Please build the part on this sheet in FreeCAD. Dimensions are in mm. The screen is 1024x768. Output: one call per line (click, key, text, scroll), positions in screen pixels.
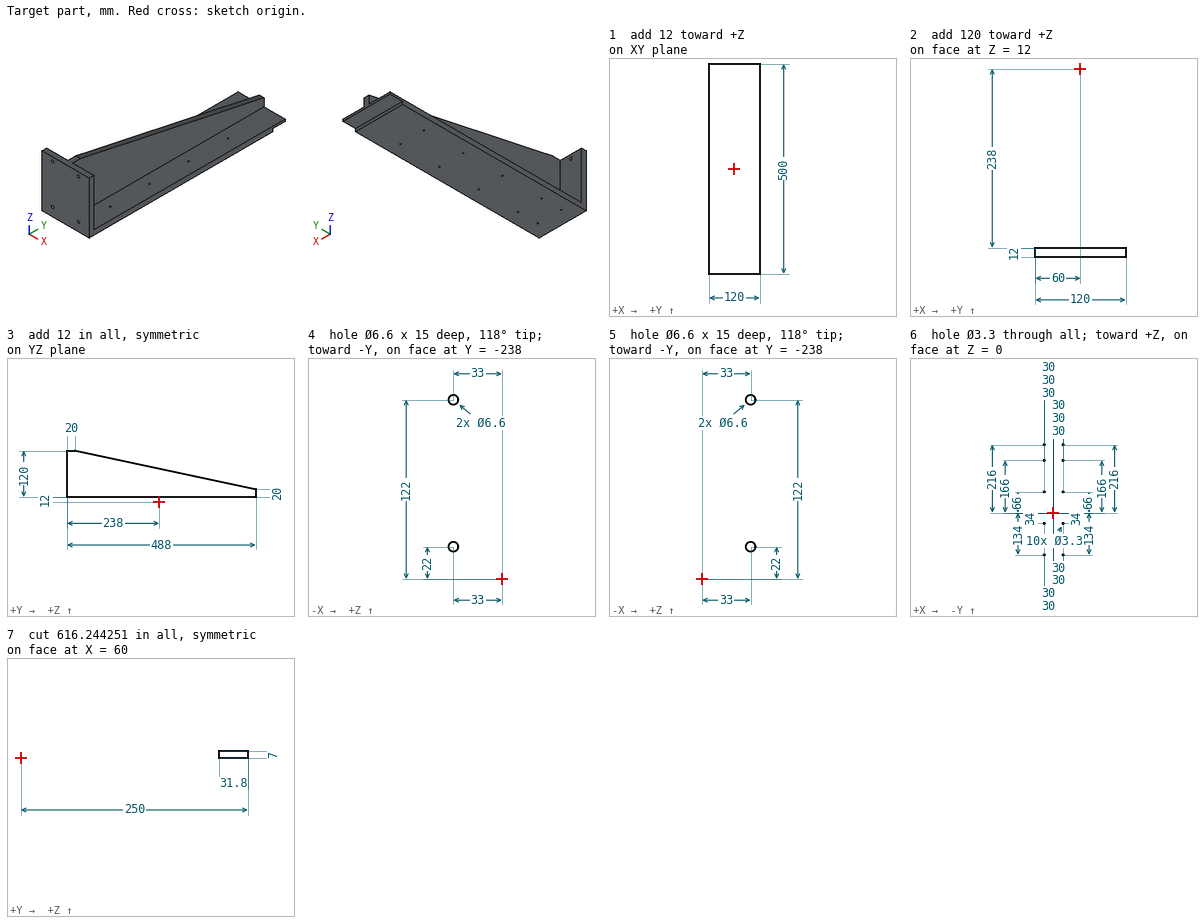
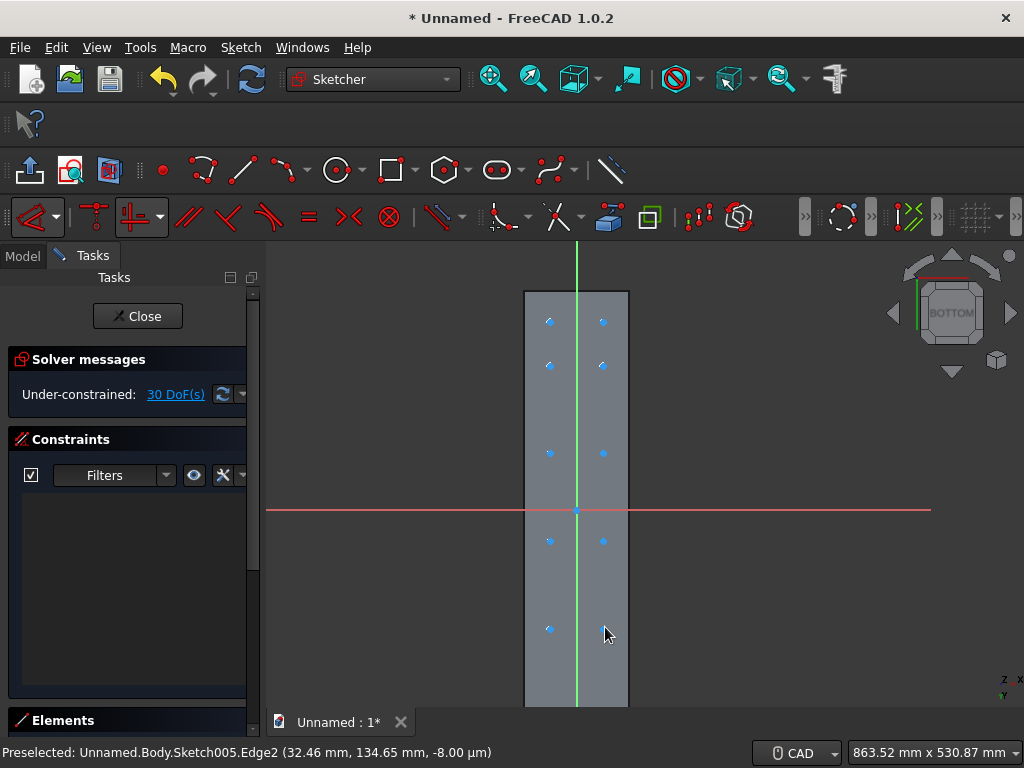
scroll(604, 452, up, 10)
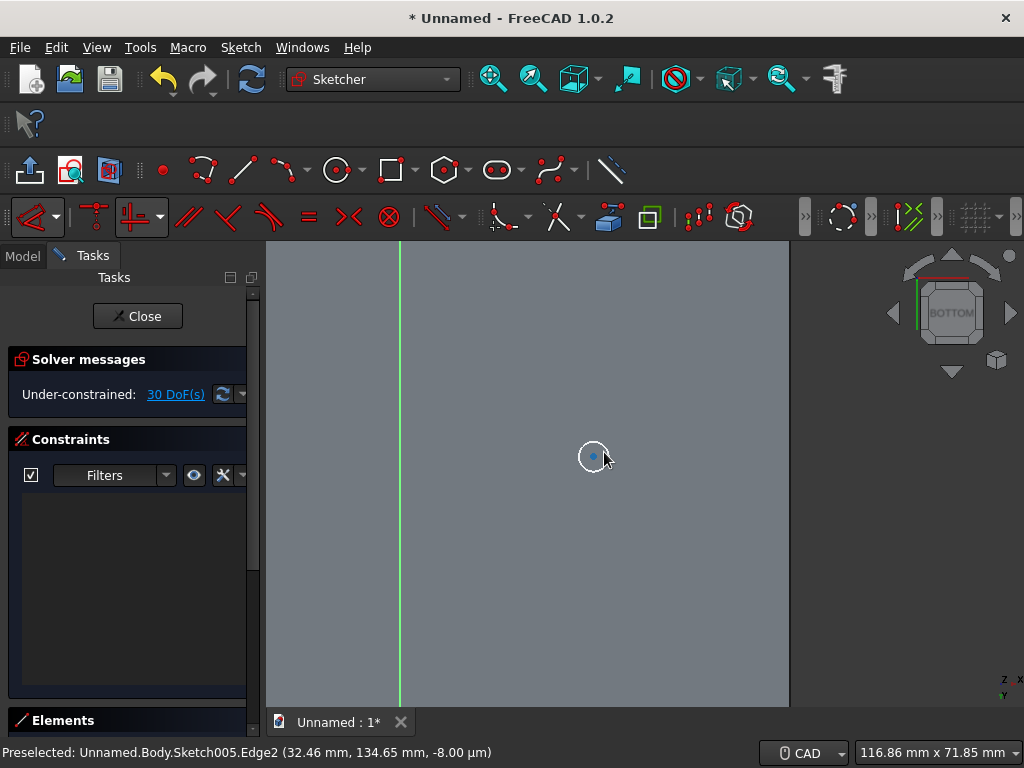
click(604, 446)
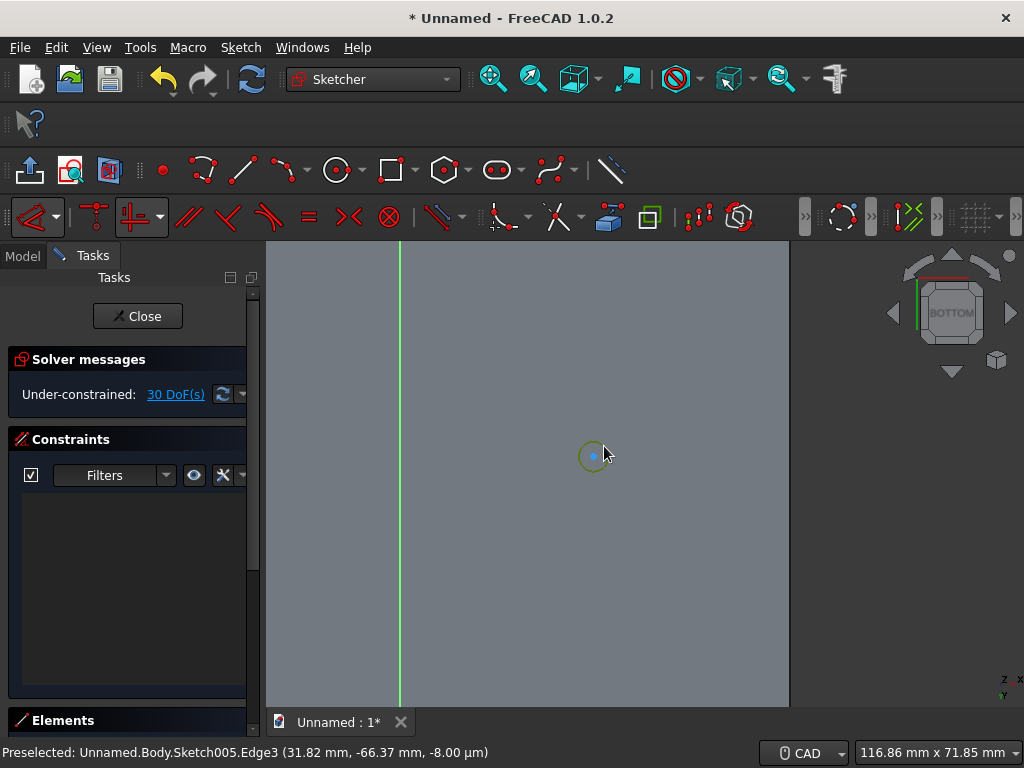
scroll(604, 452, down, 10)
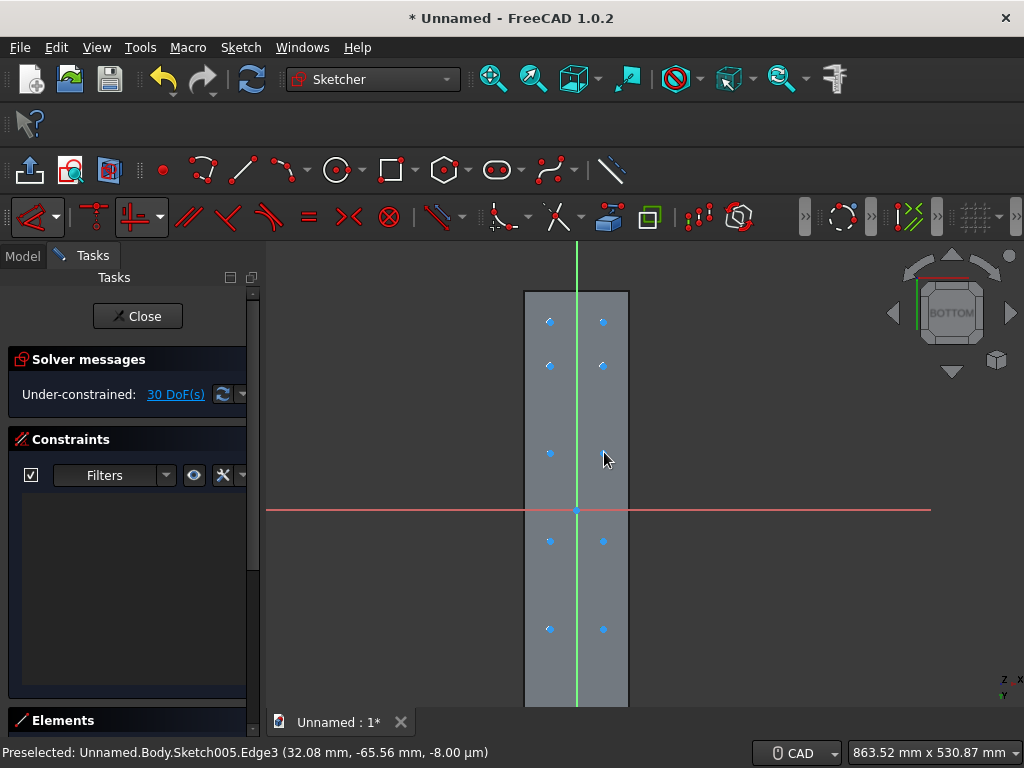
scroll(605, 364, up, 9)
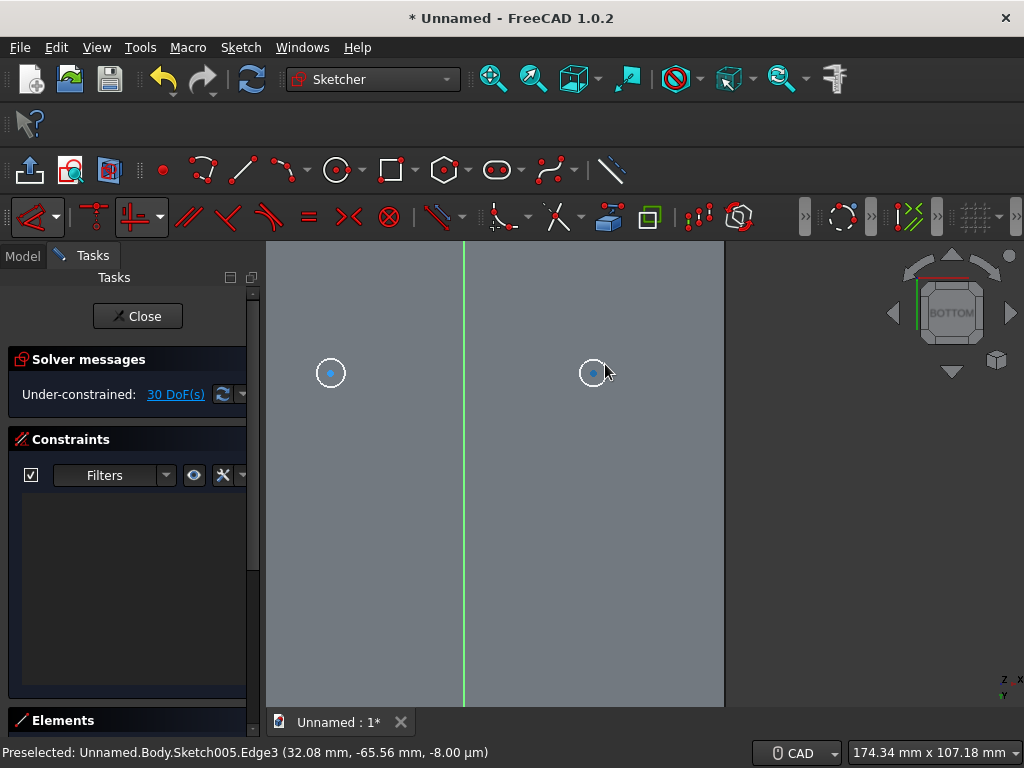
click(602, 363)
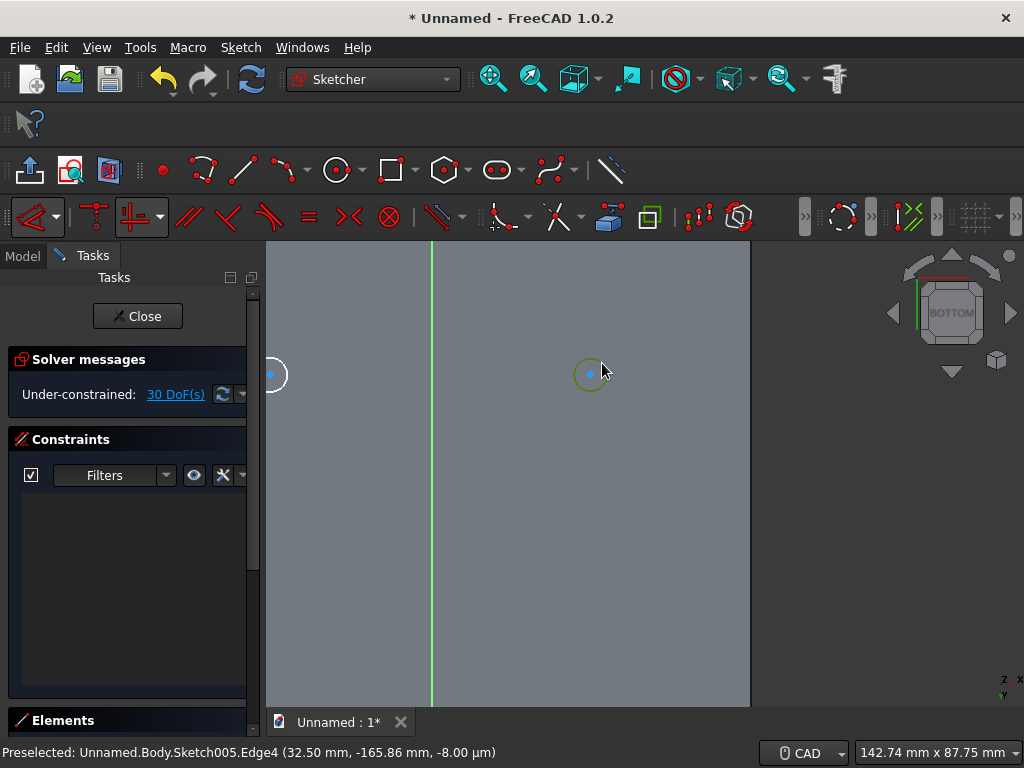
scroll(605, 364, down, 9)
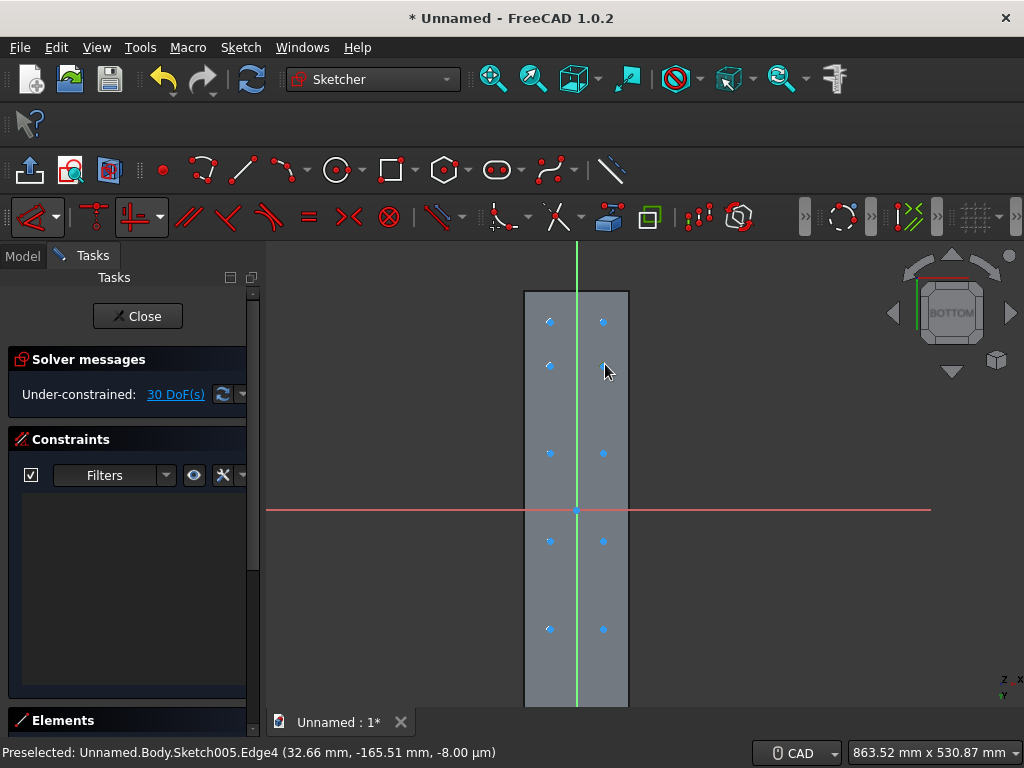
scroll(605, 320, up, 9)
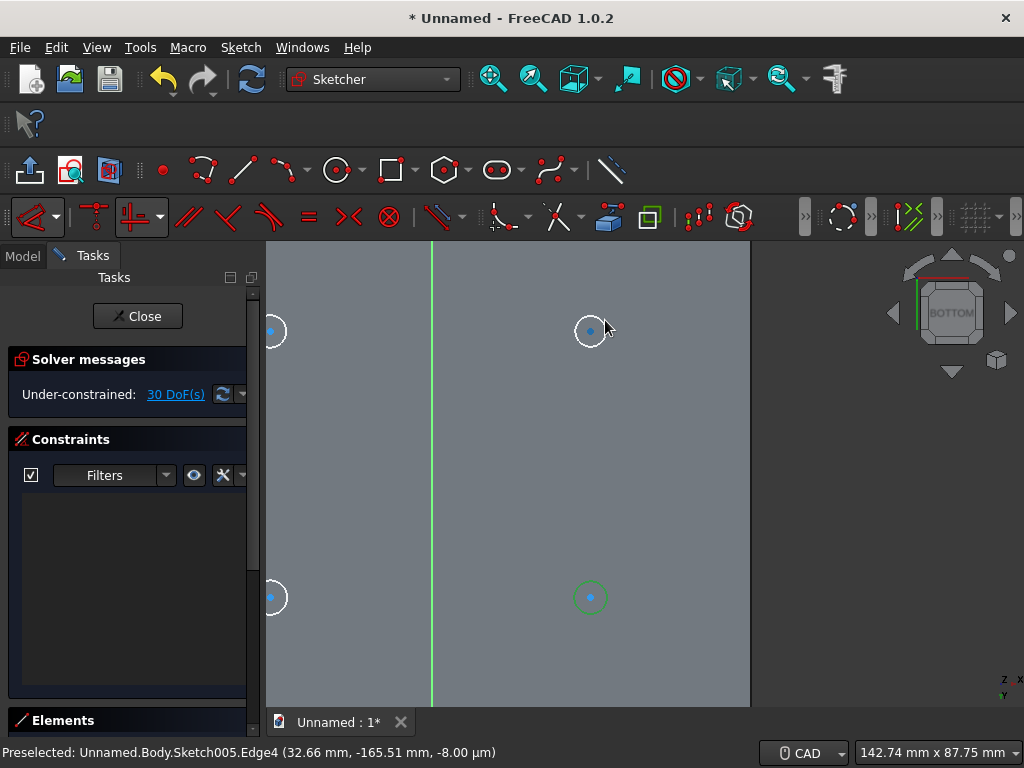
click(601, 321)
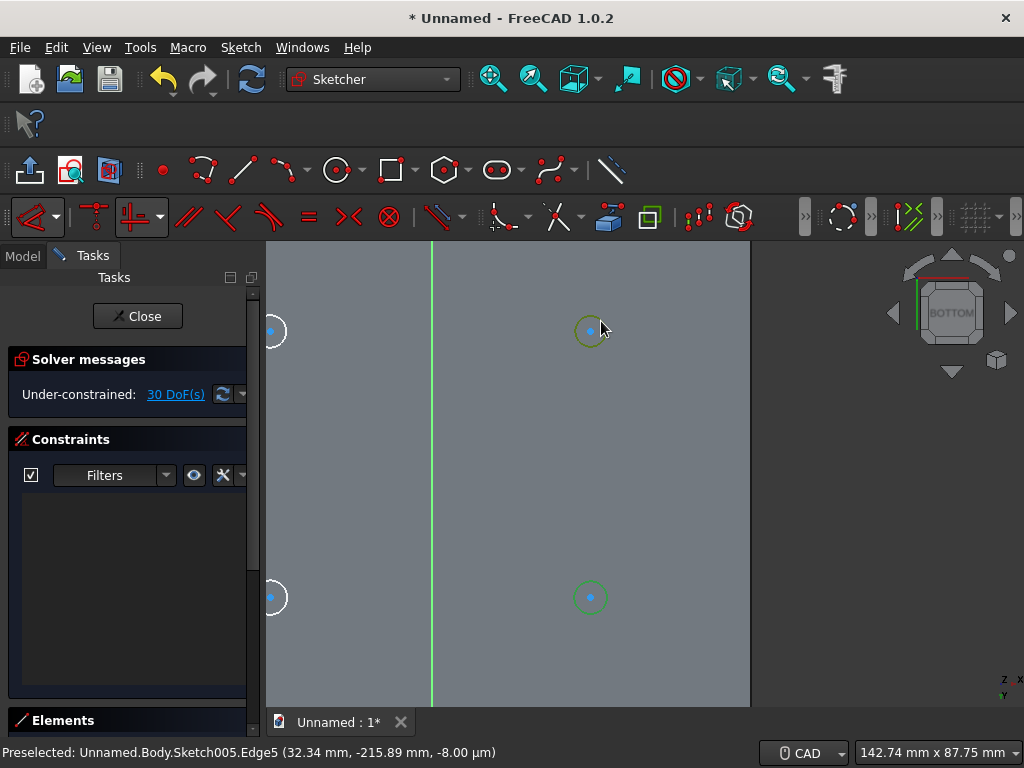
scroll(605, 320, down, 9)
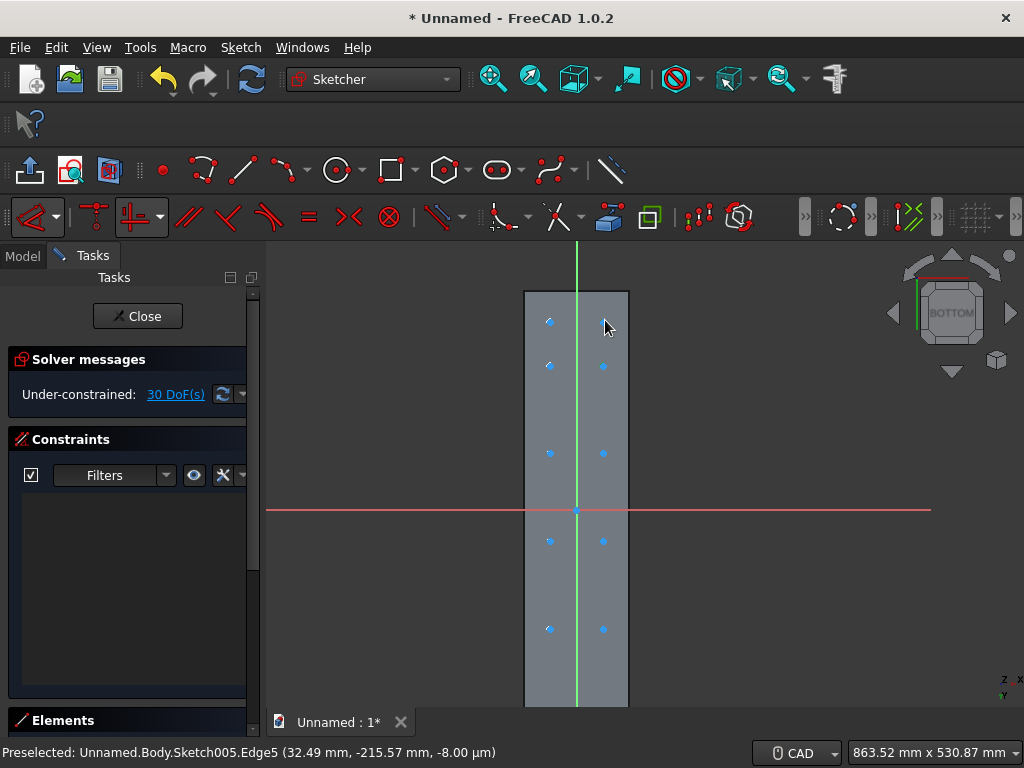
scroll(552, 320, up, 9)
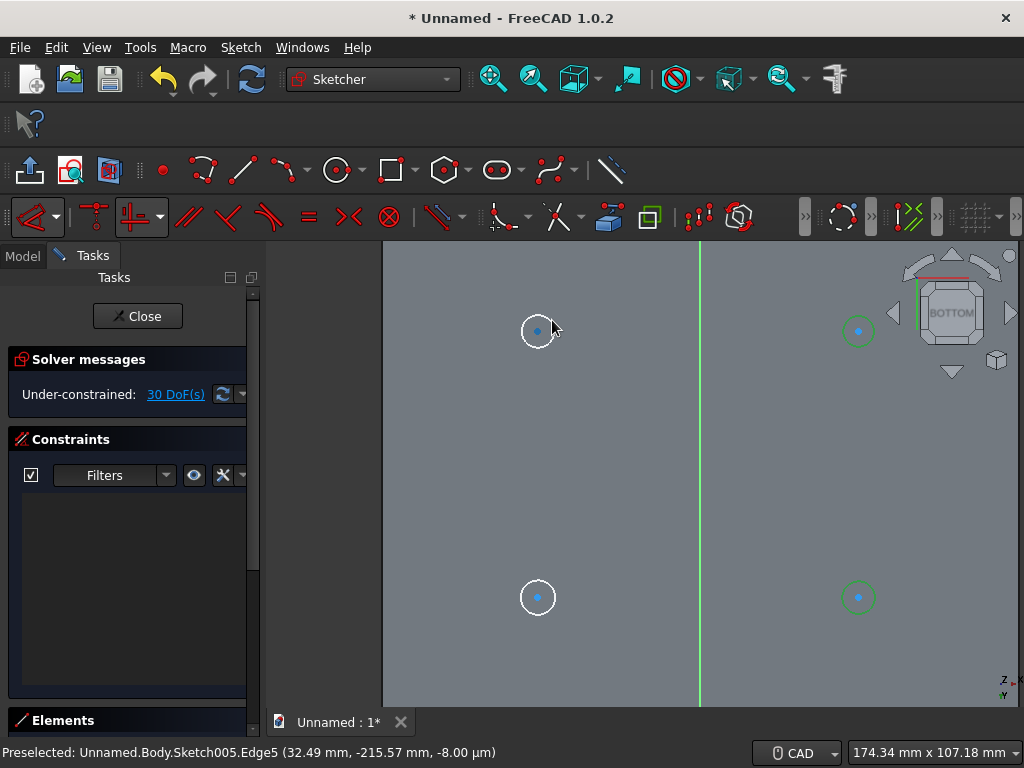
click(549, 320)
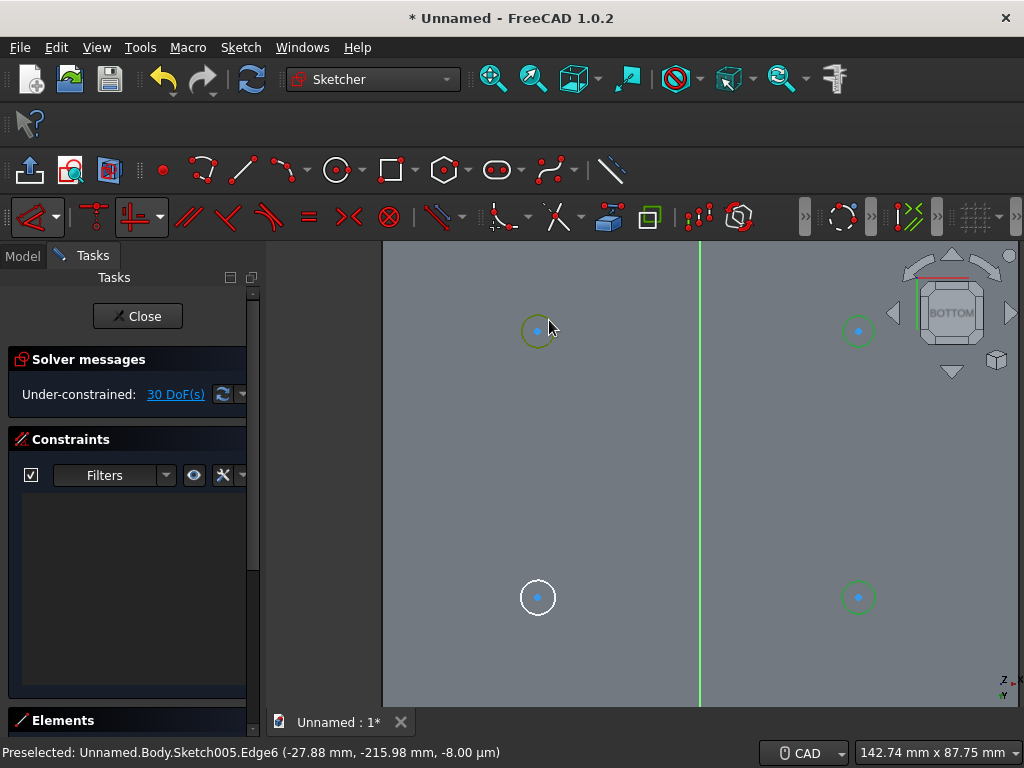
click(550, 585)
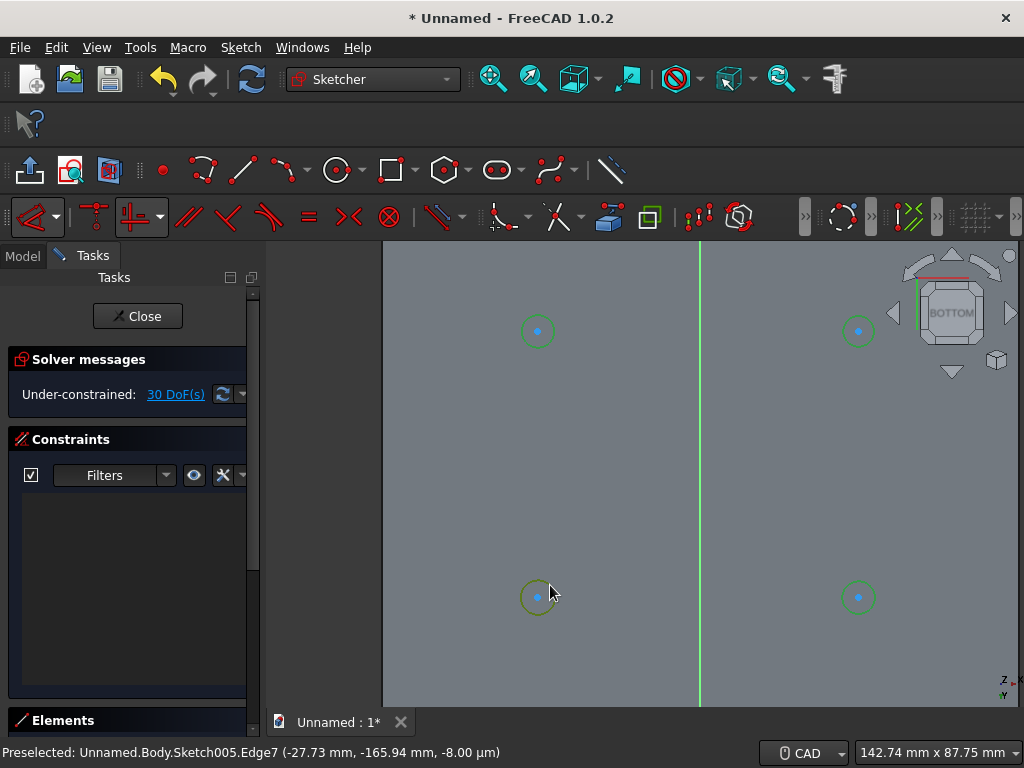
scroll(552, 320, down, 9)